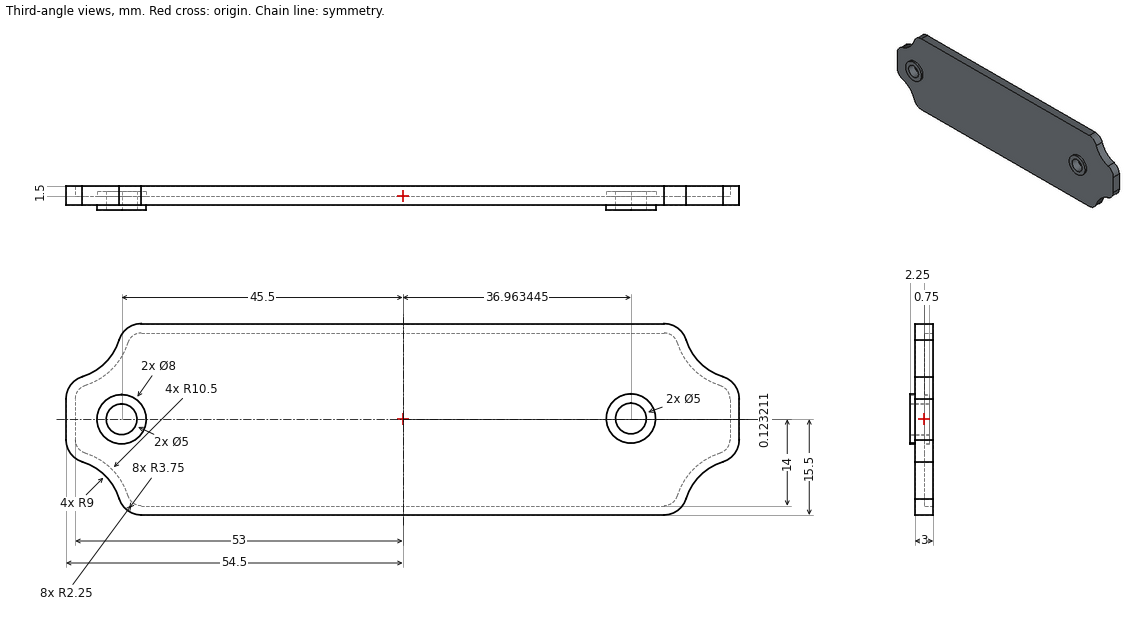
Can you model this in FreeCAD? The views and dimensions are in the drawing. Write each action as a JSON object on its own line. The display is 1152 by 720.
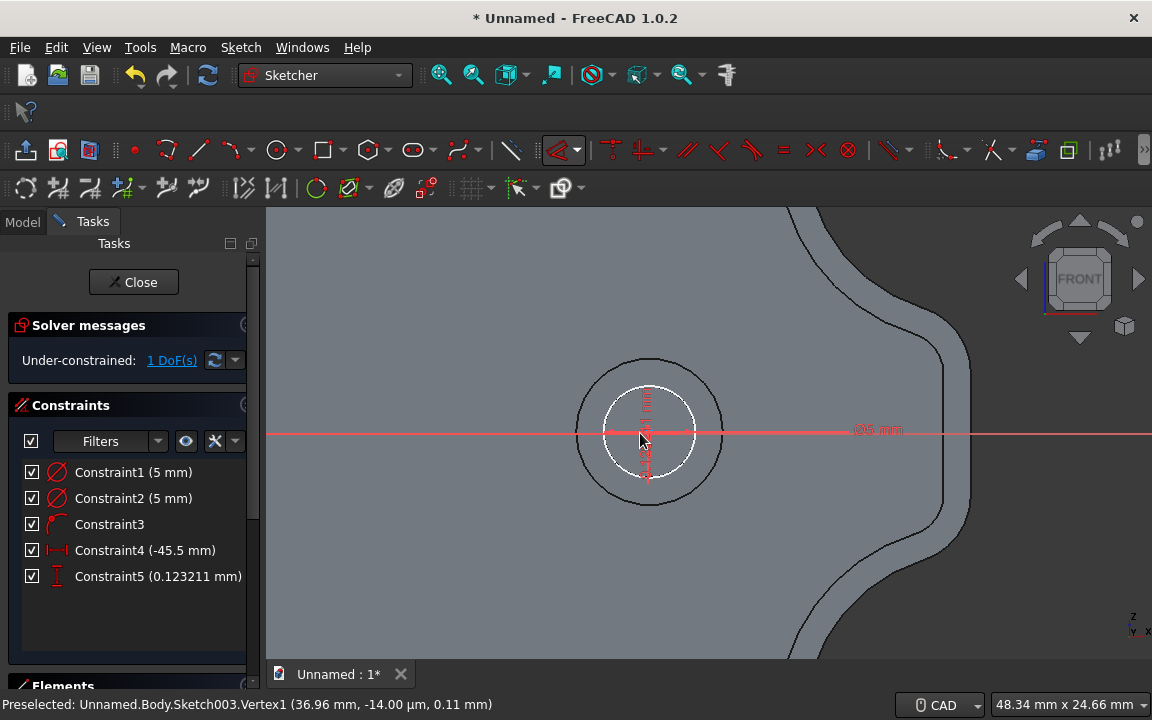
{"action": "scroll", "coordinate": [962, 433], "scroll_direction": "down", "scroll_amount": 6}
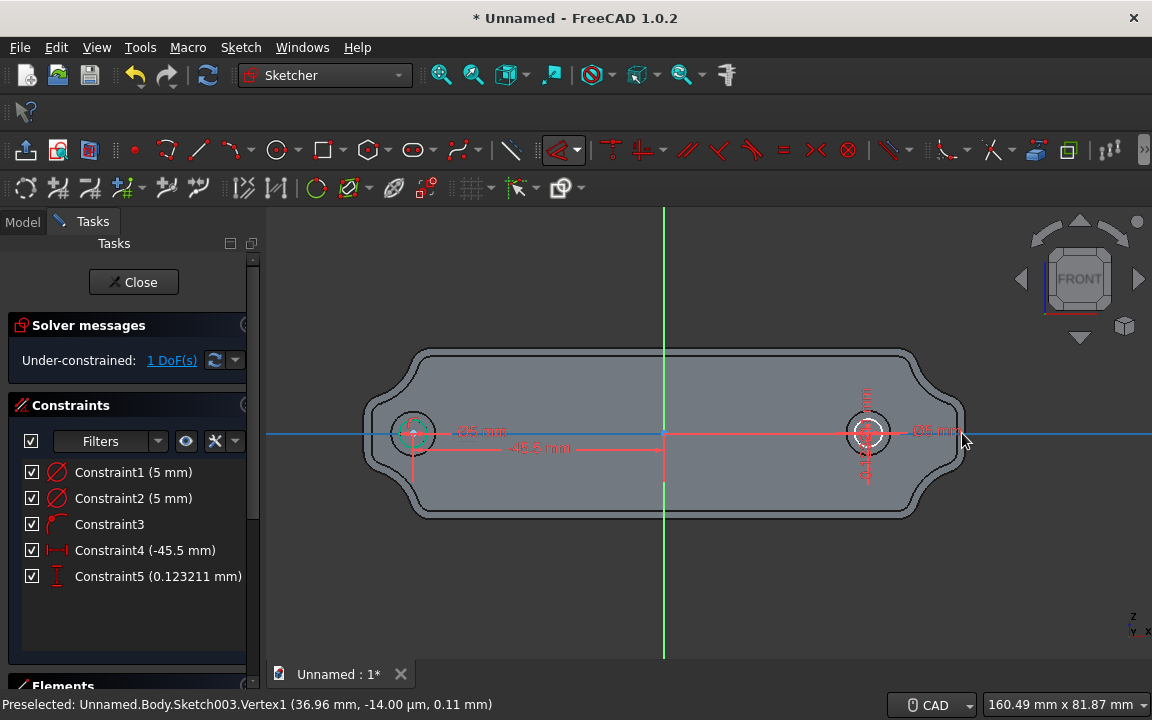
{"action": "left_click", "coordinate": [868, 433]}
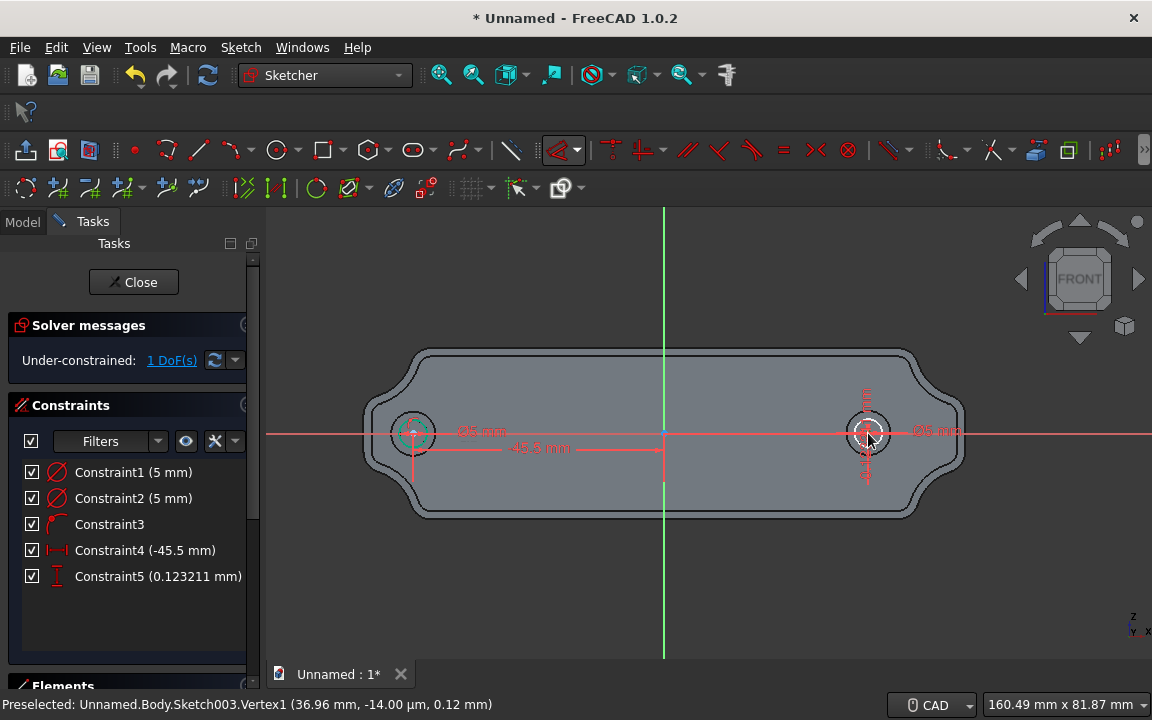
{"action": "left_click", "coordinate": [580, 150]}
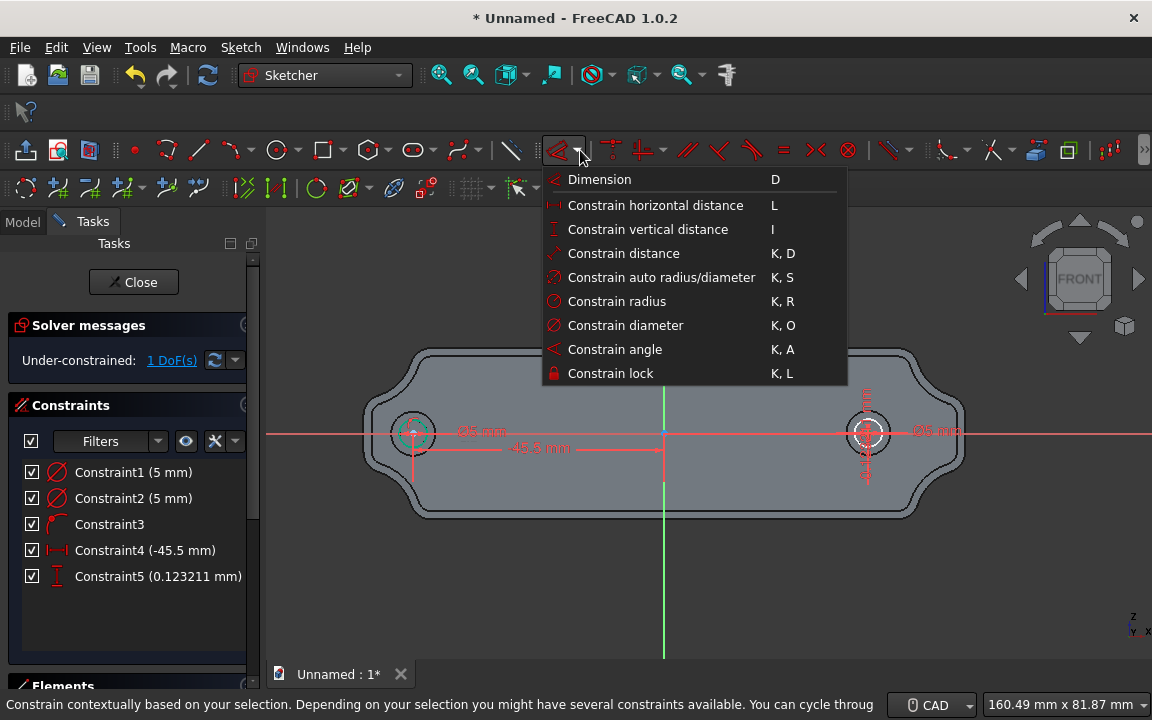
{"action": "left_click", "coordinate": [695, 205]}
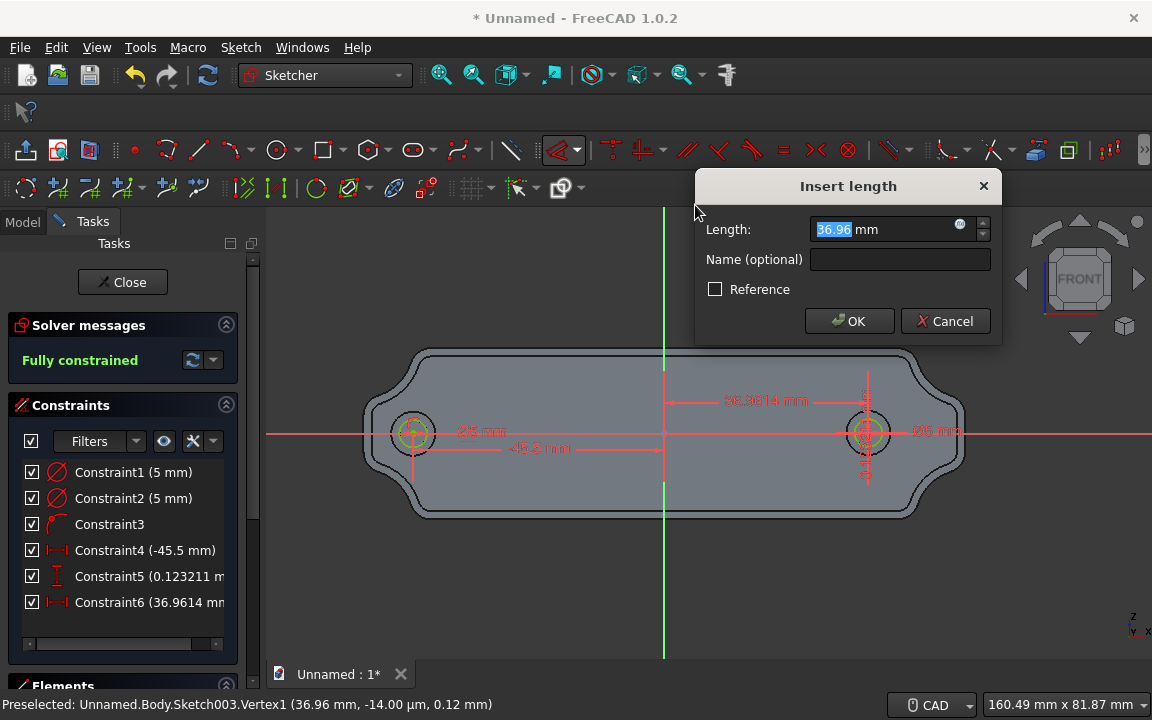
{"action": "type", "text": "36.963445"}
{"action": "key", "text": "Return"}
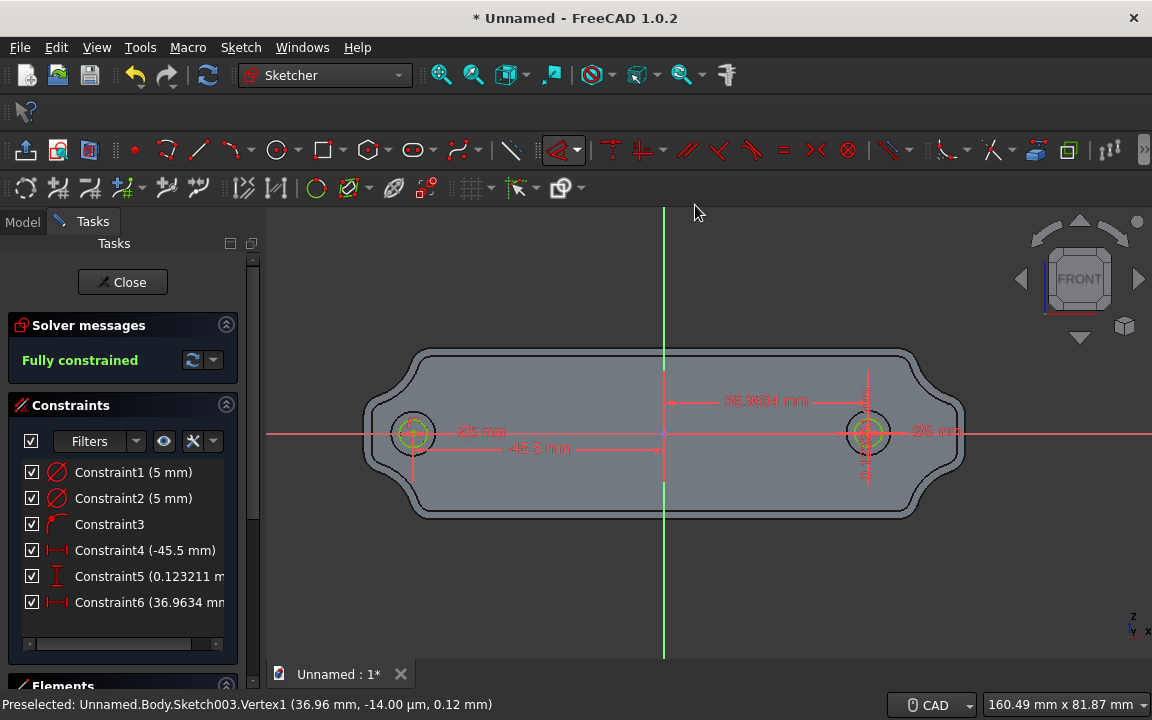
{"action": "left_click", "coordinate": [123, 282]}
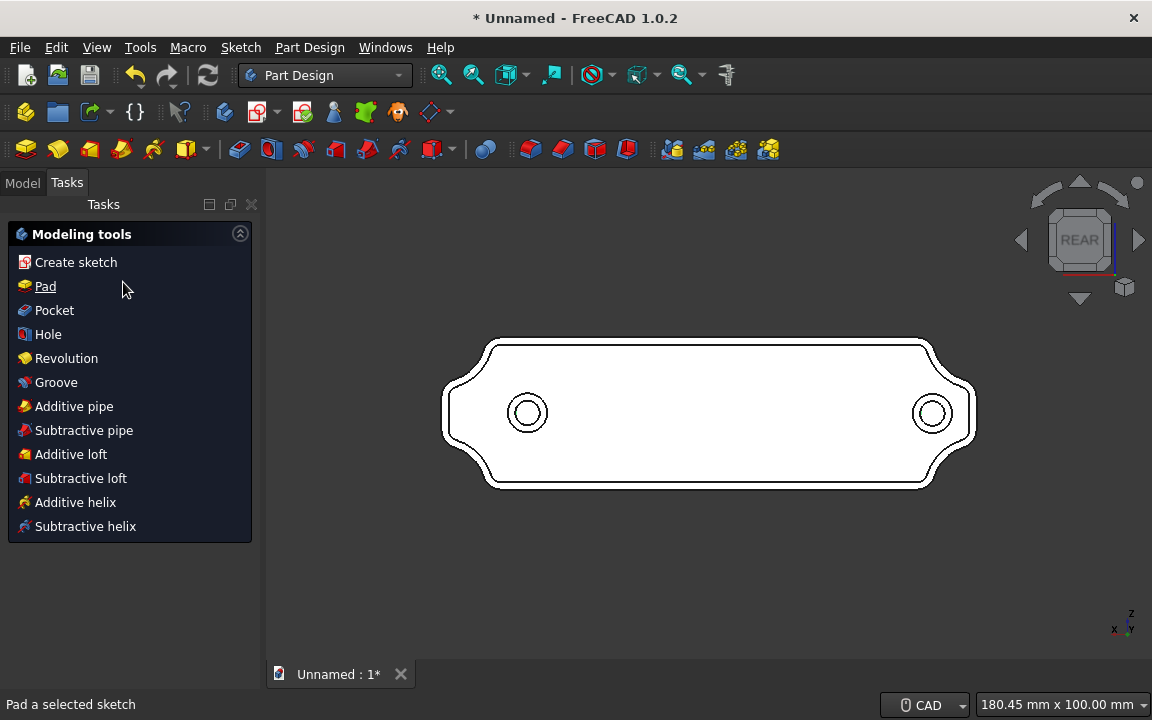
{"action": "left_click", "coordinate": [240, 150]}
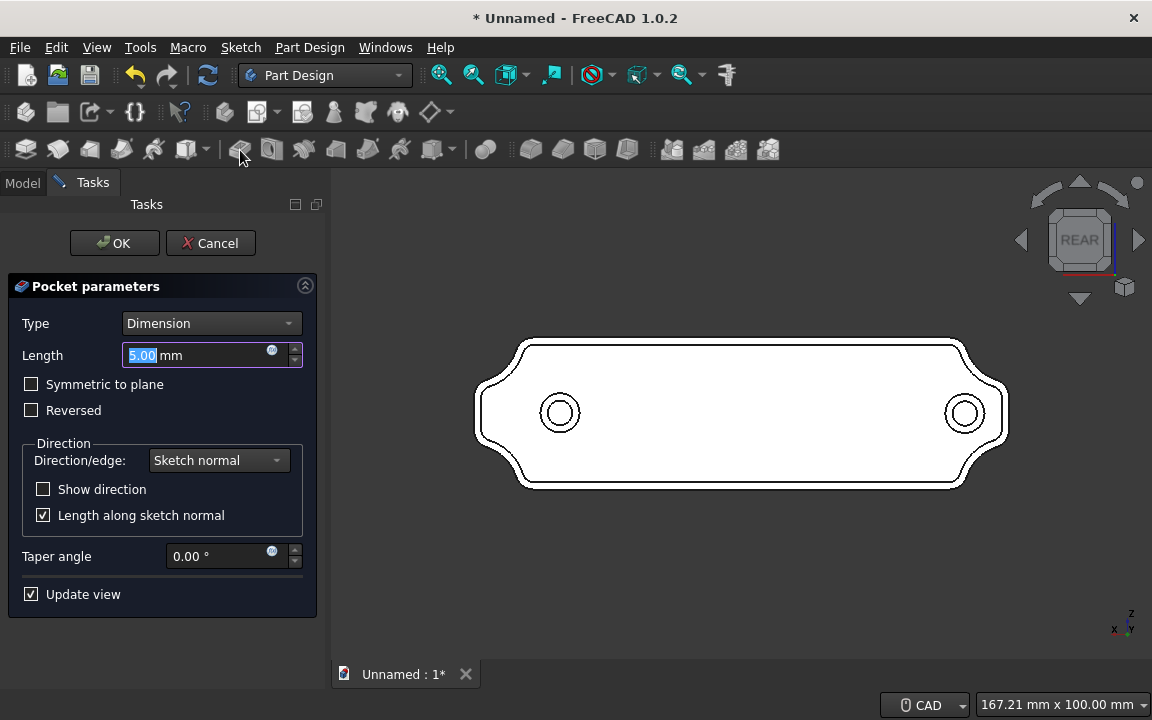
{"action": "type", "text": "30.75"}
{"action": "key", "text": "Tab"}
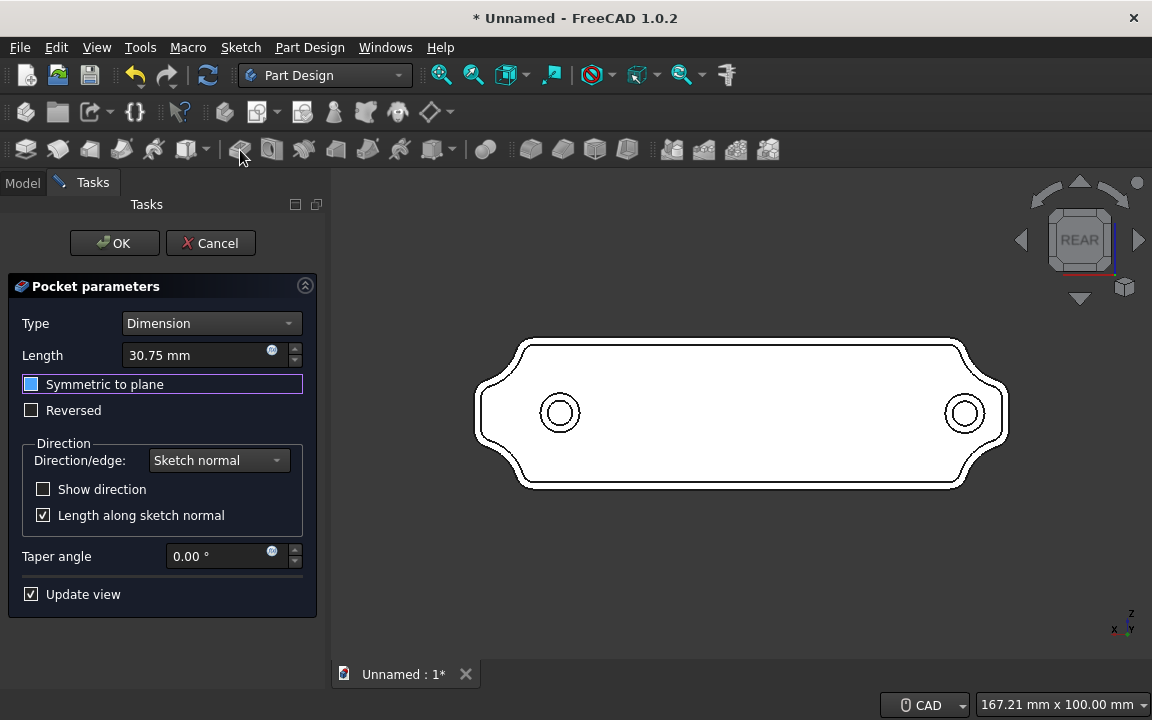
{"action": "left_click", "coordinate": [30, 410]}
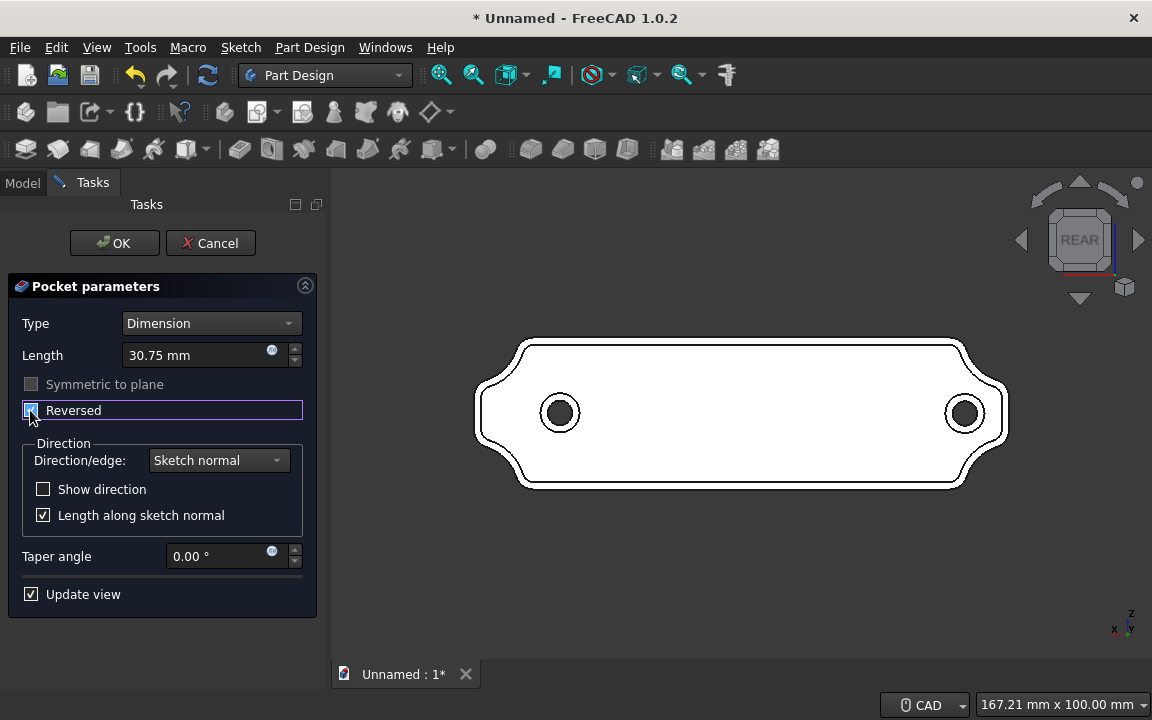
{"action": "left_click", "coordinate": [115, 243]}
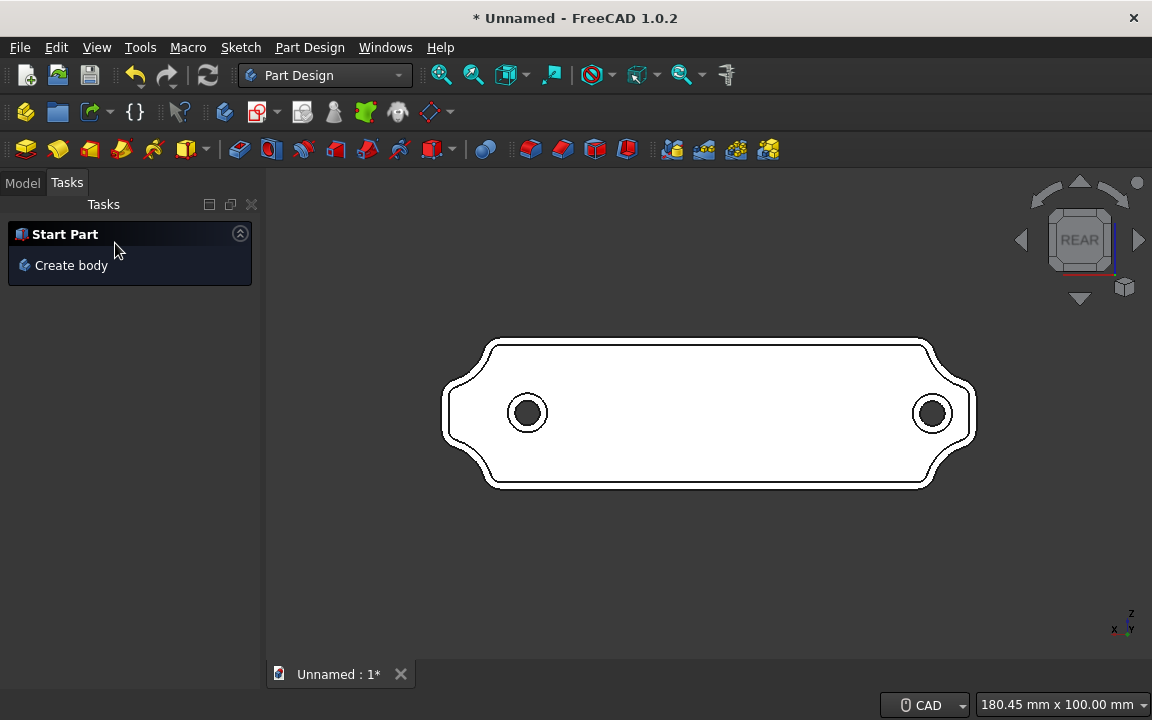
{"action": "key", "text": "0"}